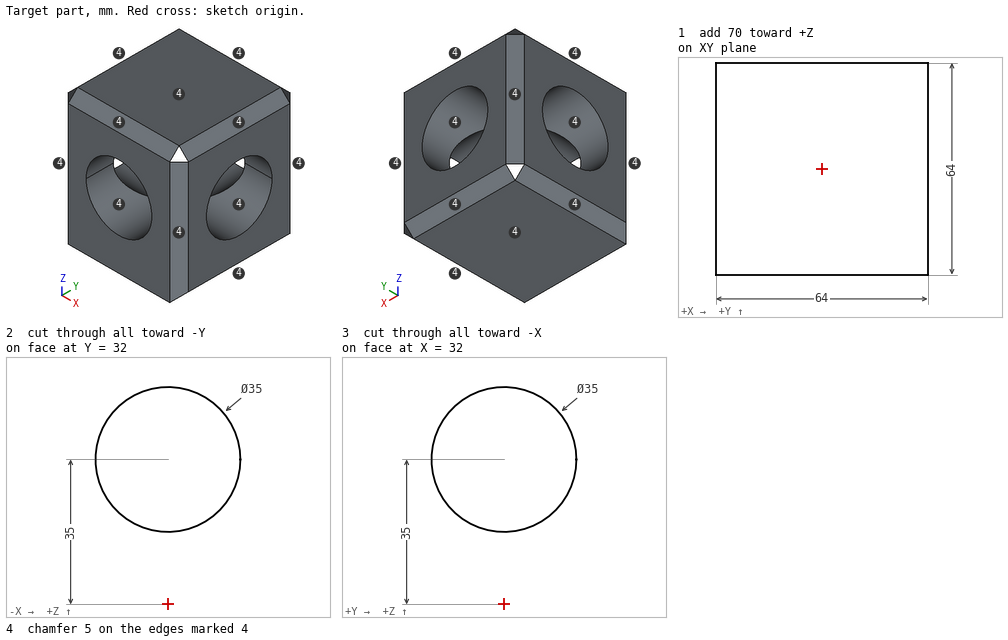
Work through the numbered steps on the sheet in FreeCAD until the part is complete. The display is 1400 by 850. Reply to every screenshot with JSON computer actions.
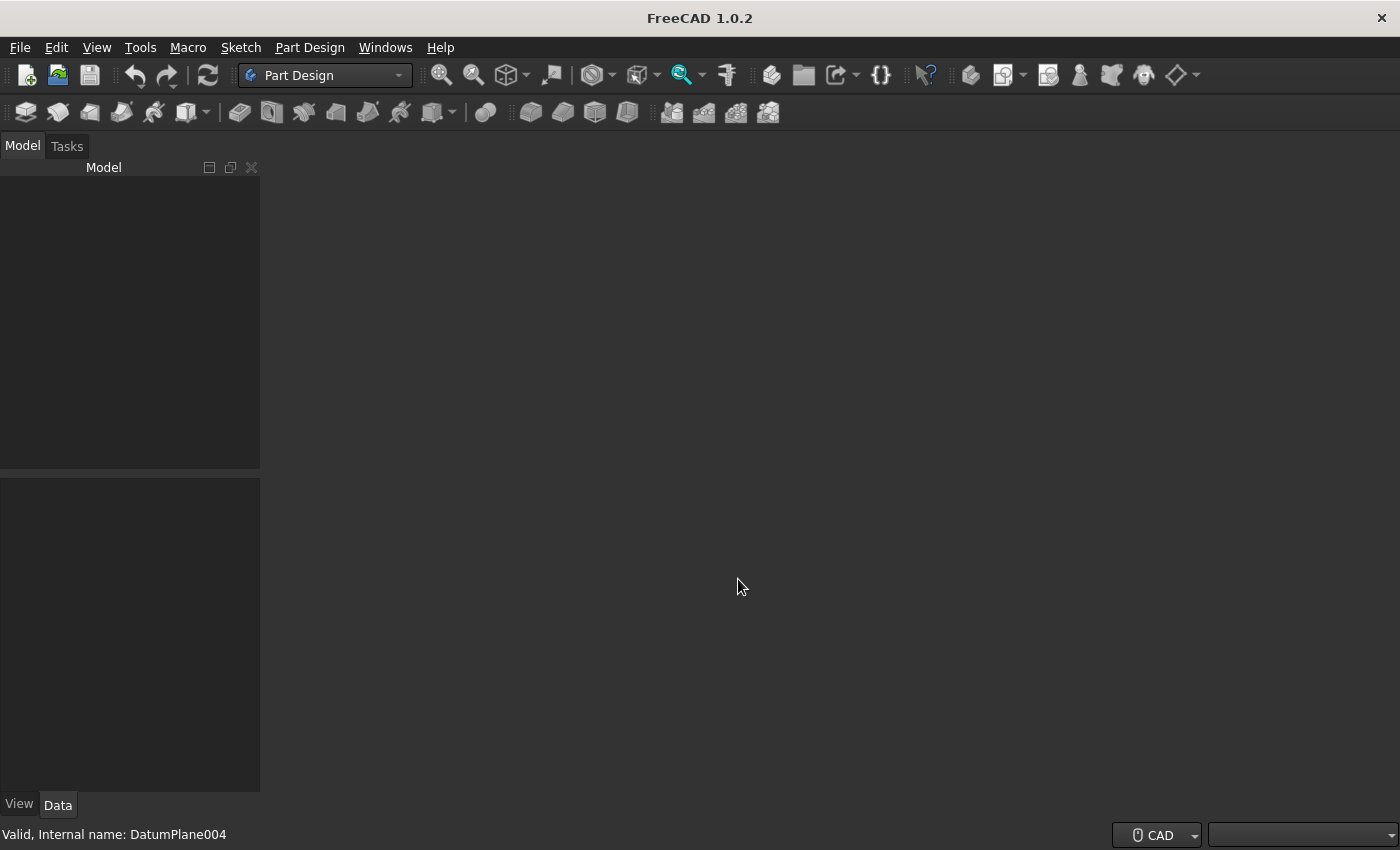
{"action": "key", "text": "ctrl+n"}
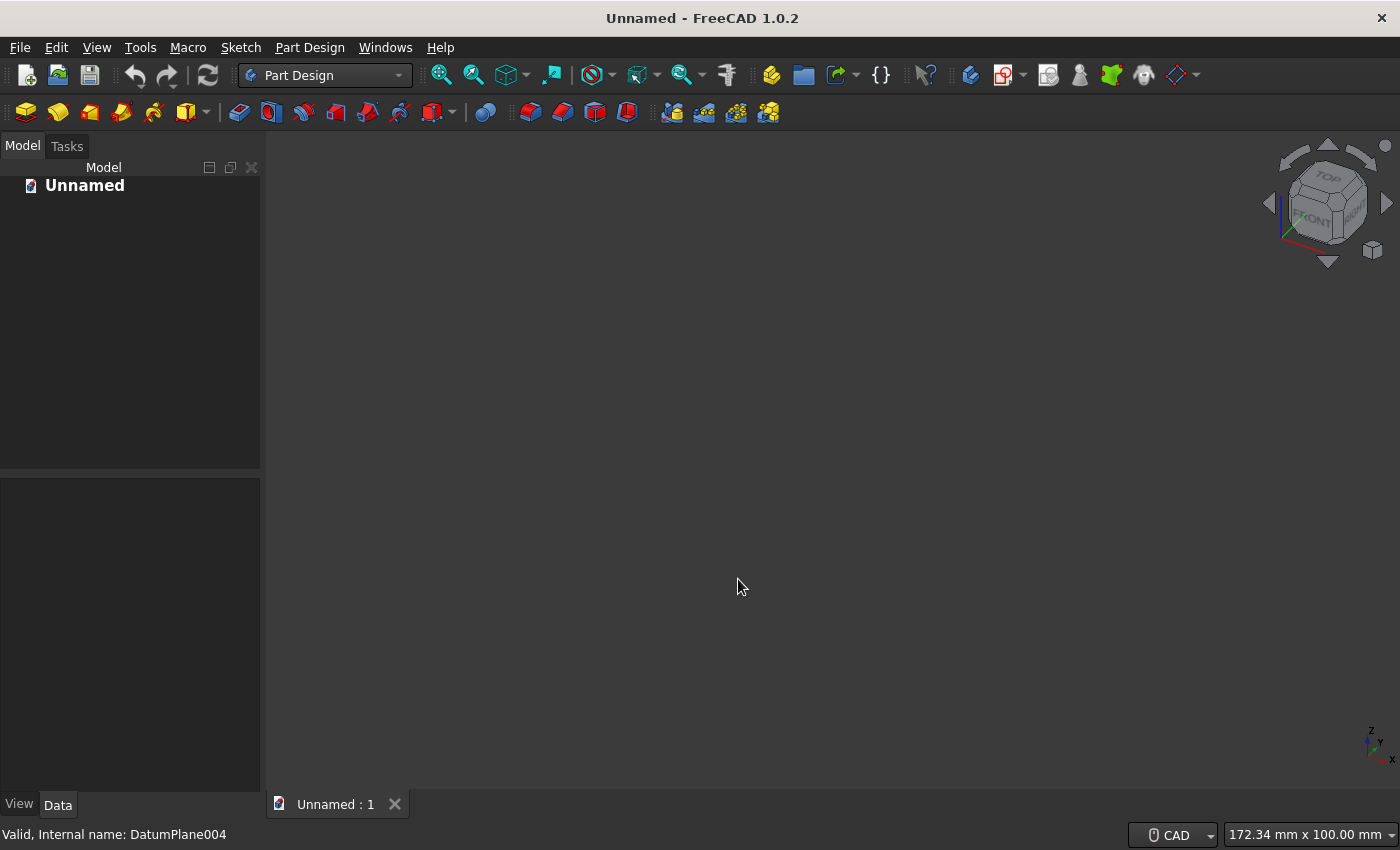
{"action": "left_click", "coordinate": [1004, 76]}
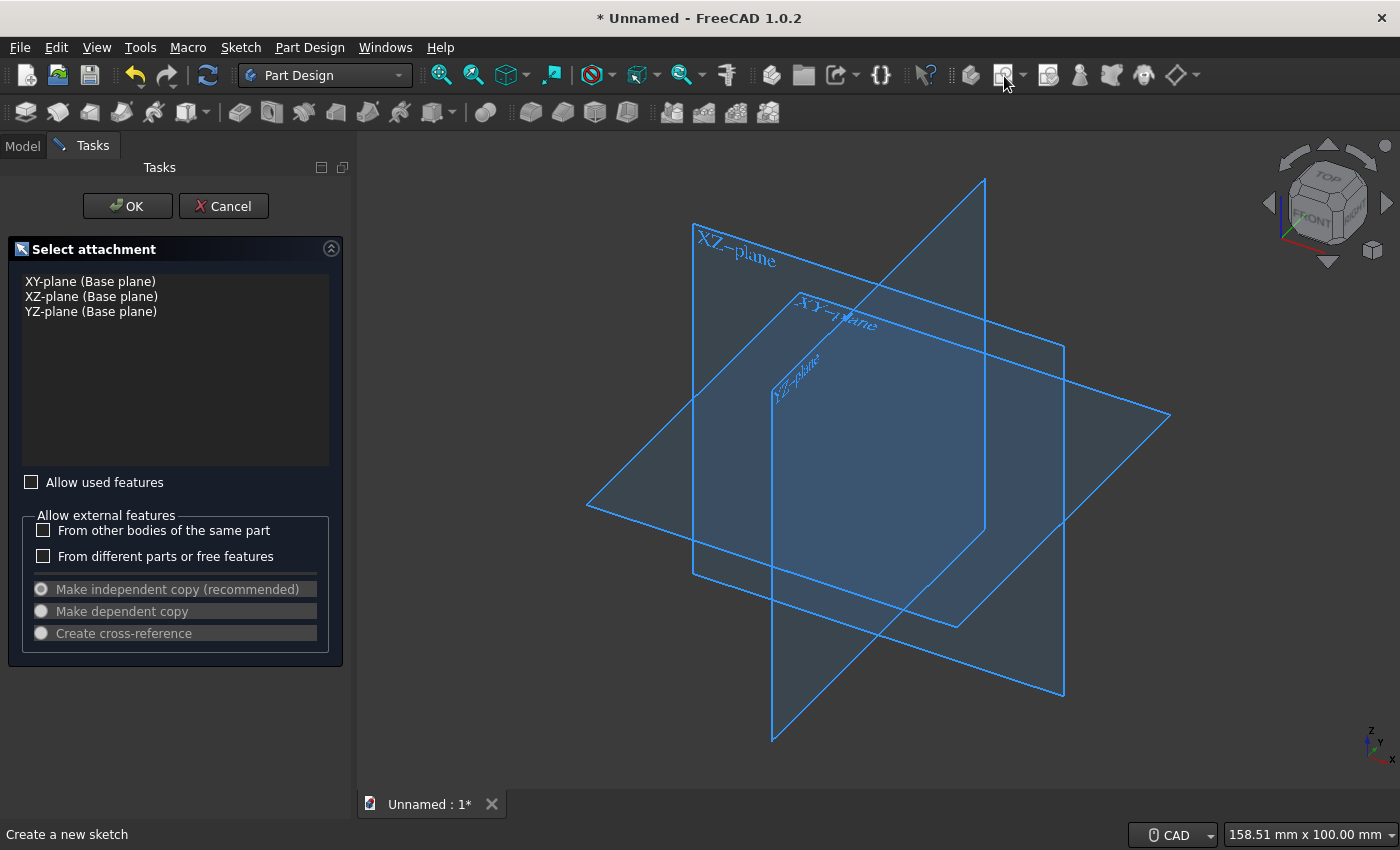
{"action": "left_click", "coordinate": [82, 282]}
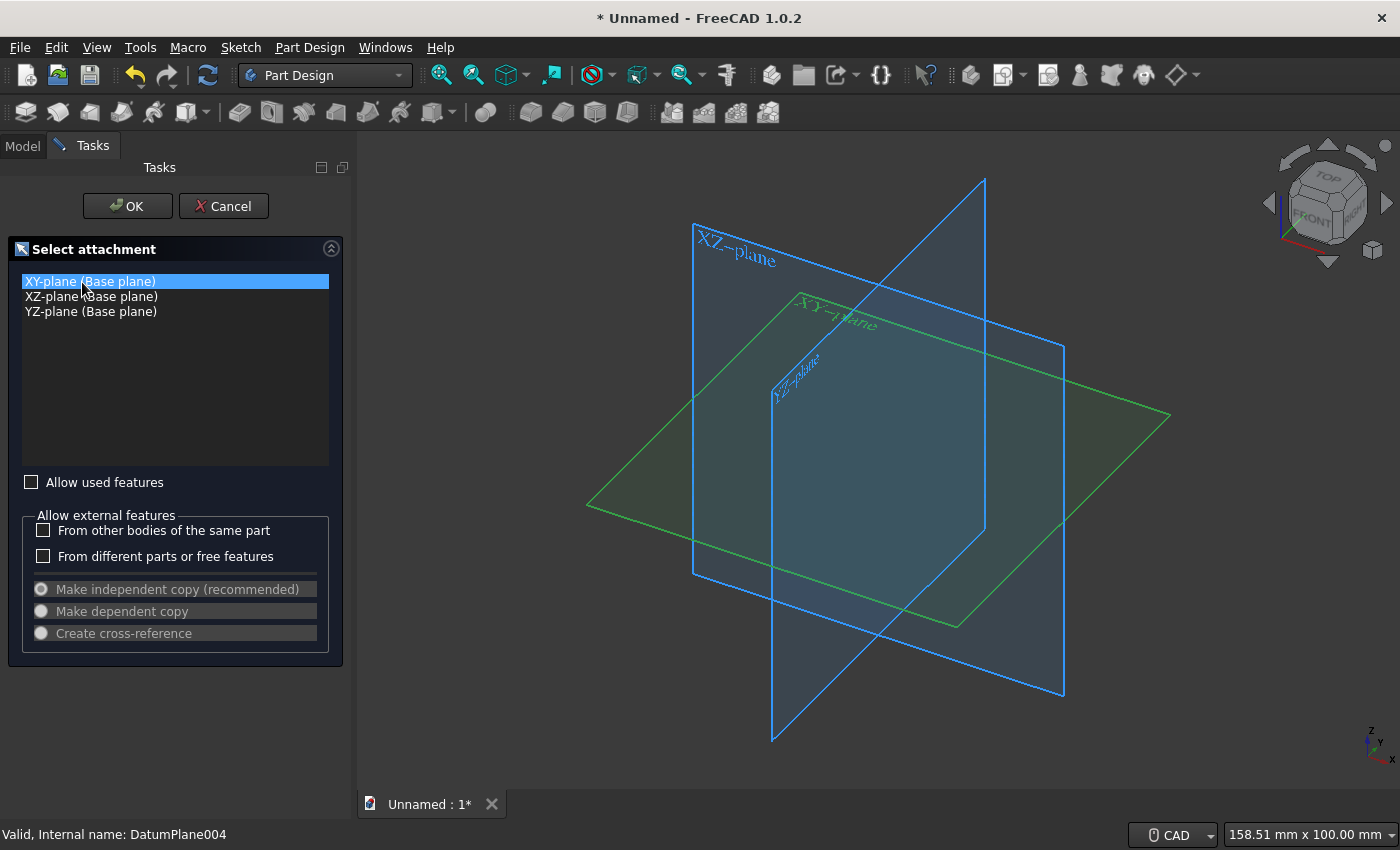
{"action": "left_click", "coordinate": [128, 206]}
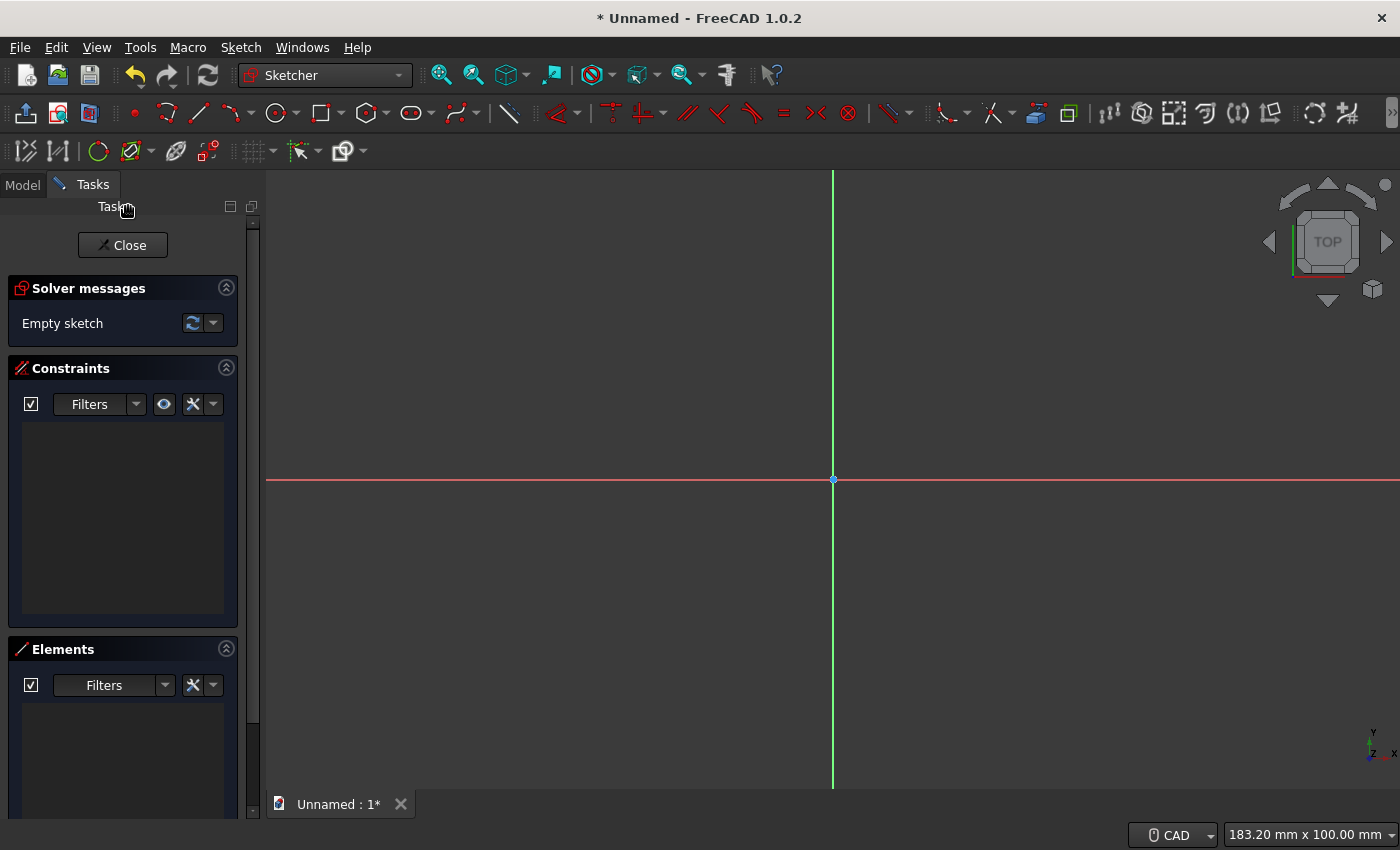
{"action": "left_click", "coordinate": [344, 114]}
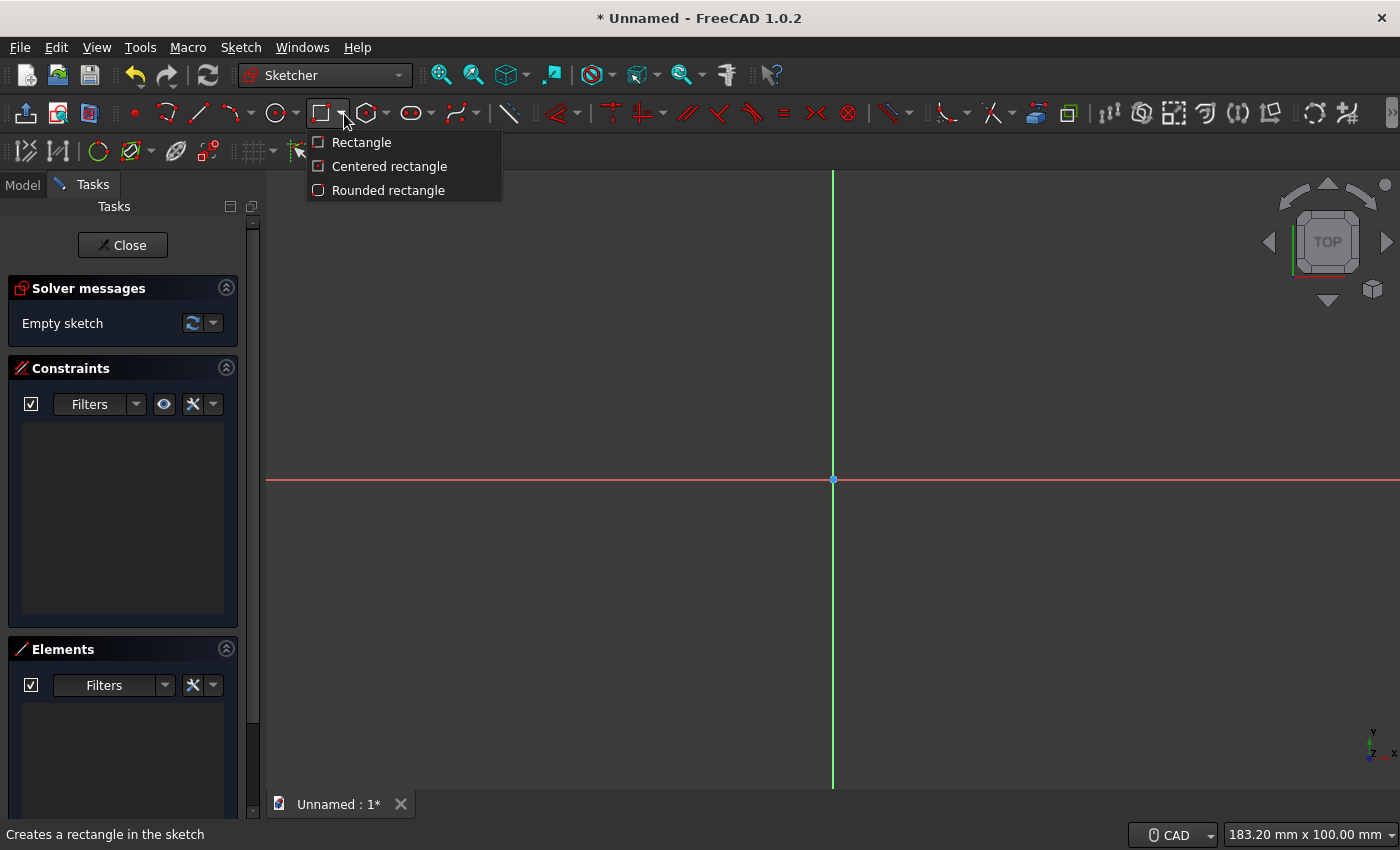
{"action": "left_click", "coordinate": [404, 166]}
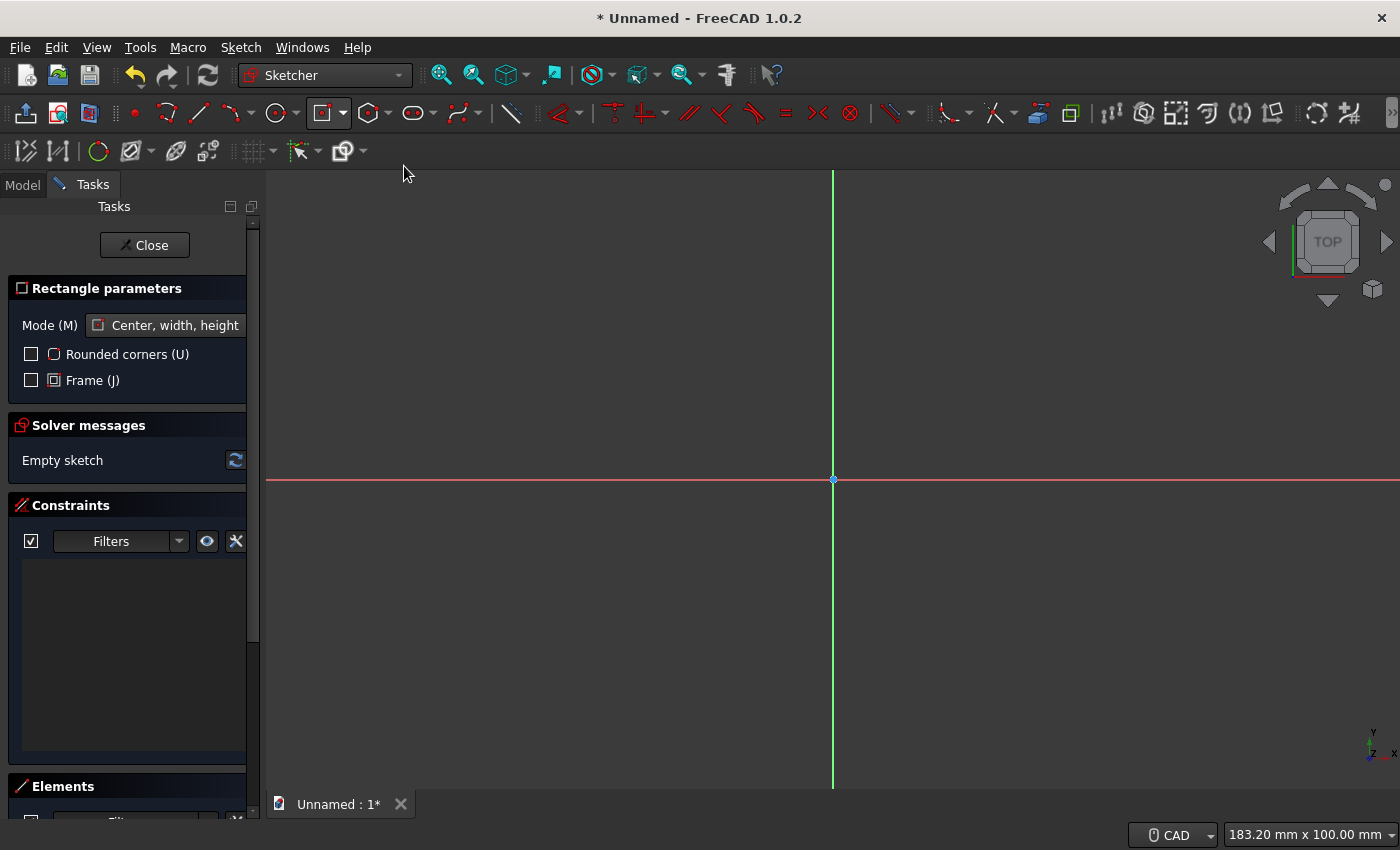
{"action": "left_click", "coordinate": [833, 480]}
{"action": "left_click", "coordinate": [1031, 281]}
{"action": "key", "text": "Escape"}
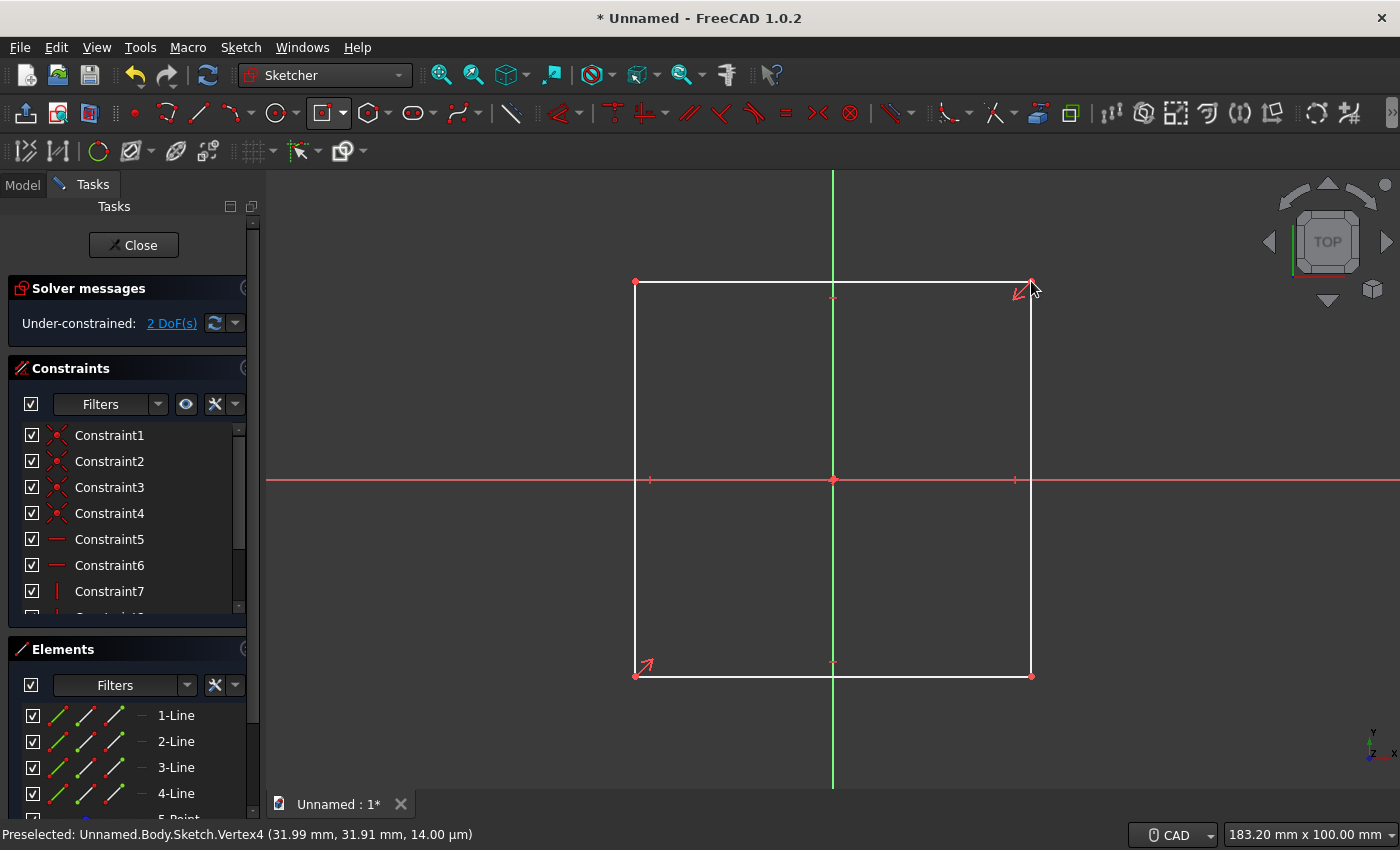
{"action": "key", "text": "d"}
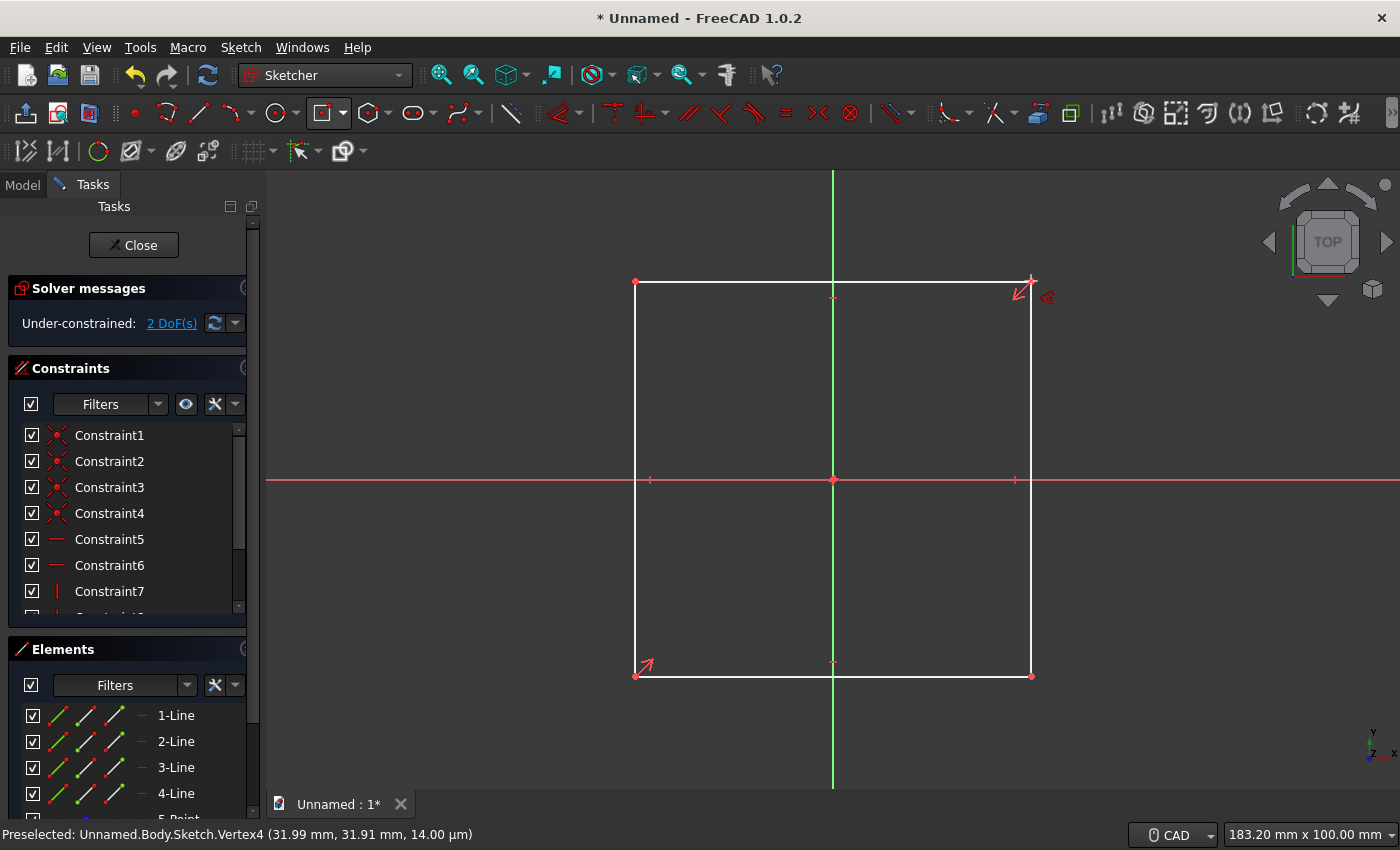
{"action": "left_click", "coordinate": [754, 677]}
{"action": "left_click", "coordinate": [742, 711]}